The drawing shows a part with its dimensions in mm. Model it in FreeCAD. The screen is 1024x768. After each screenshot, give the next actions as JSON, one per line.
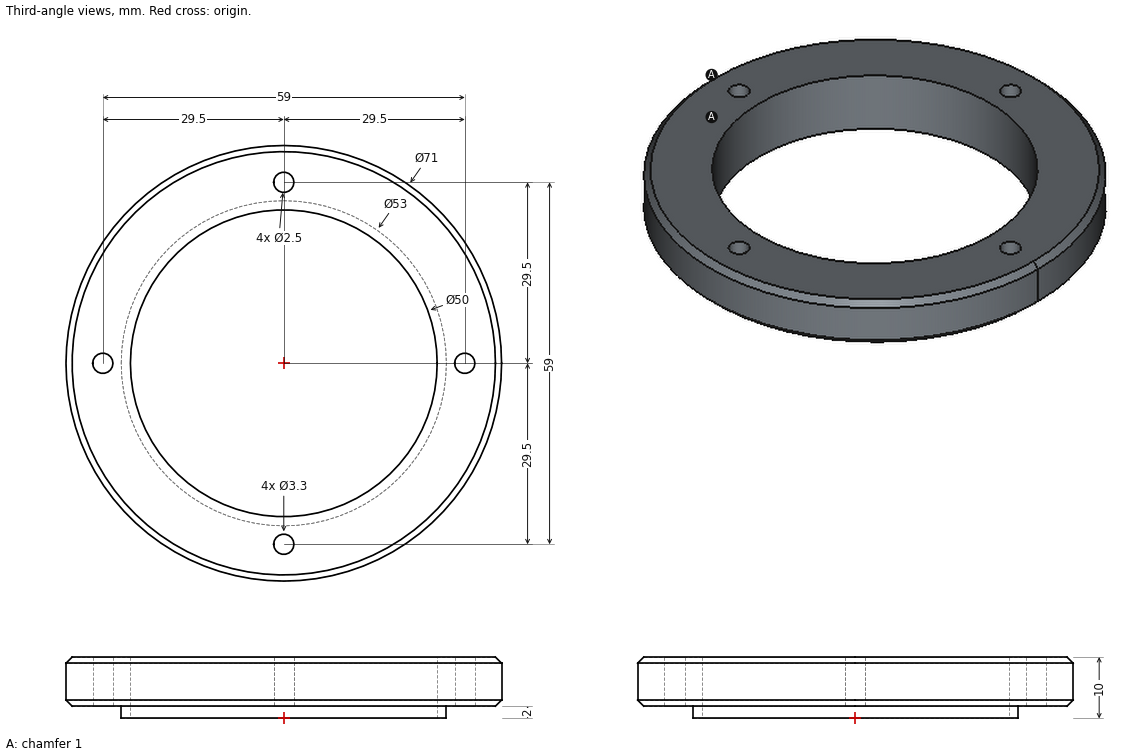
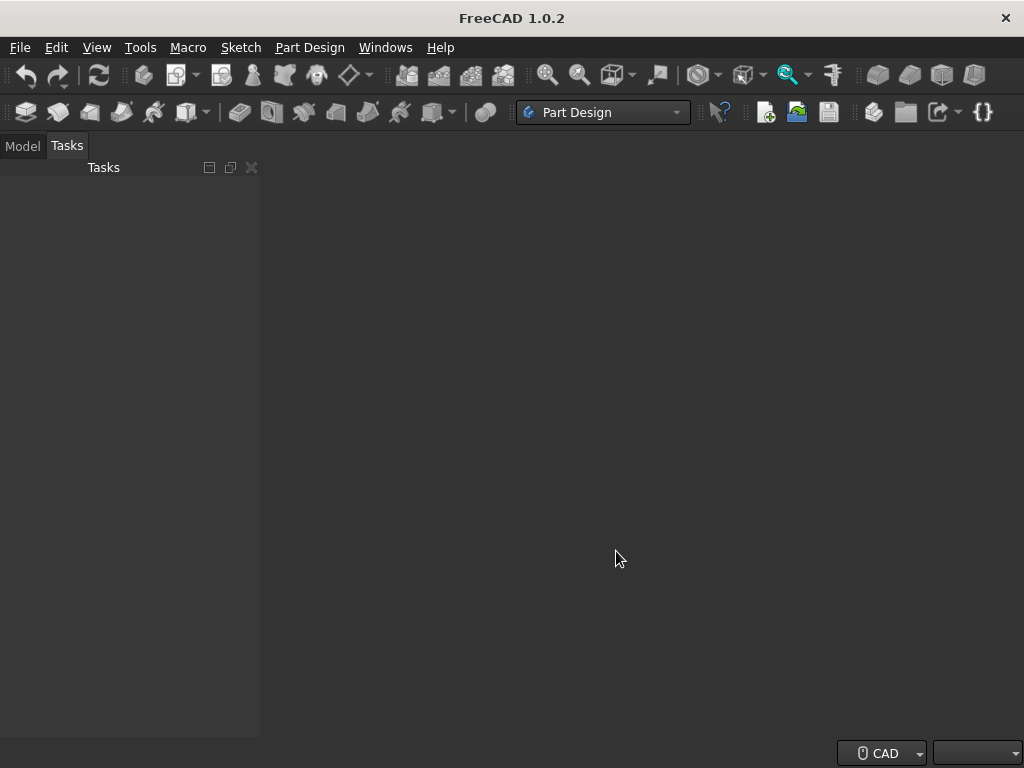
{"action": "left_click", "coordinate": [766, 112]}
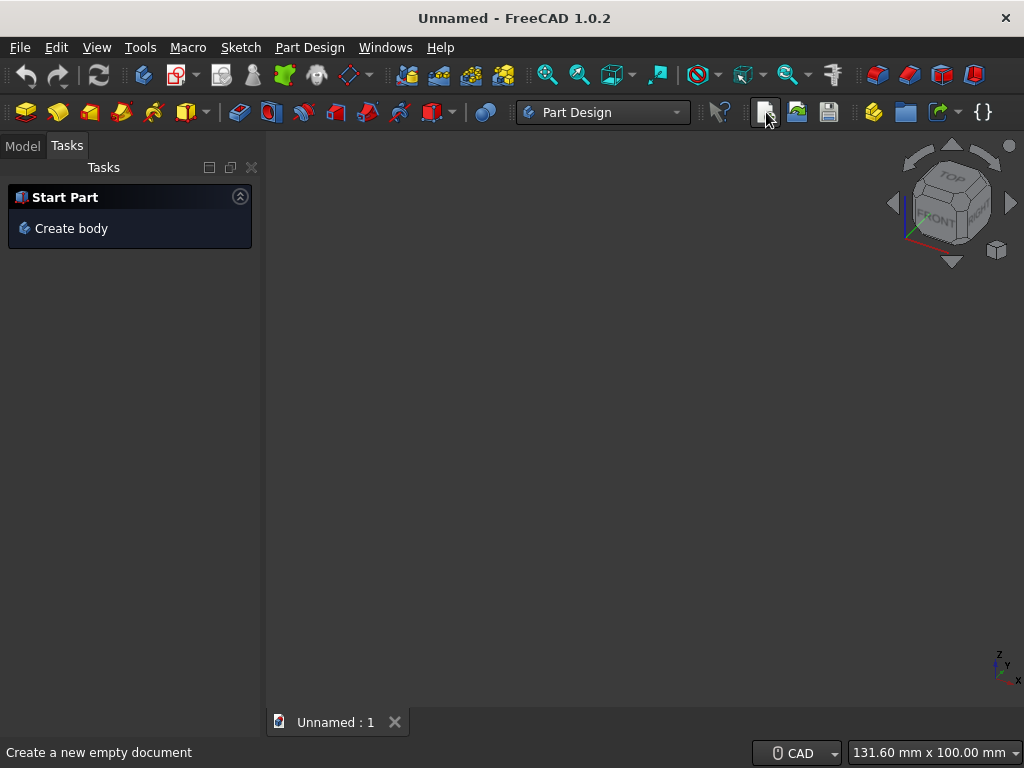
{"action": "left_click", "coordinate": [176, 76]}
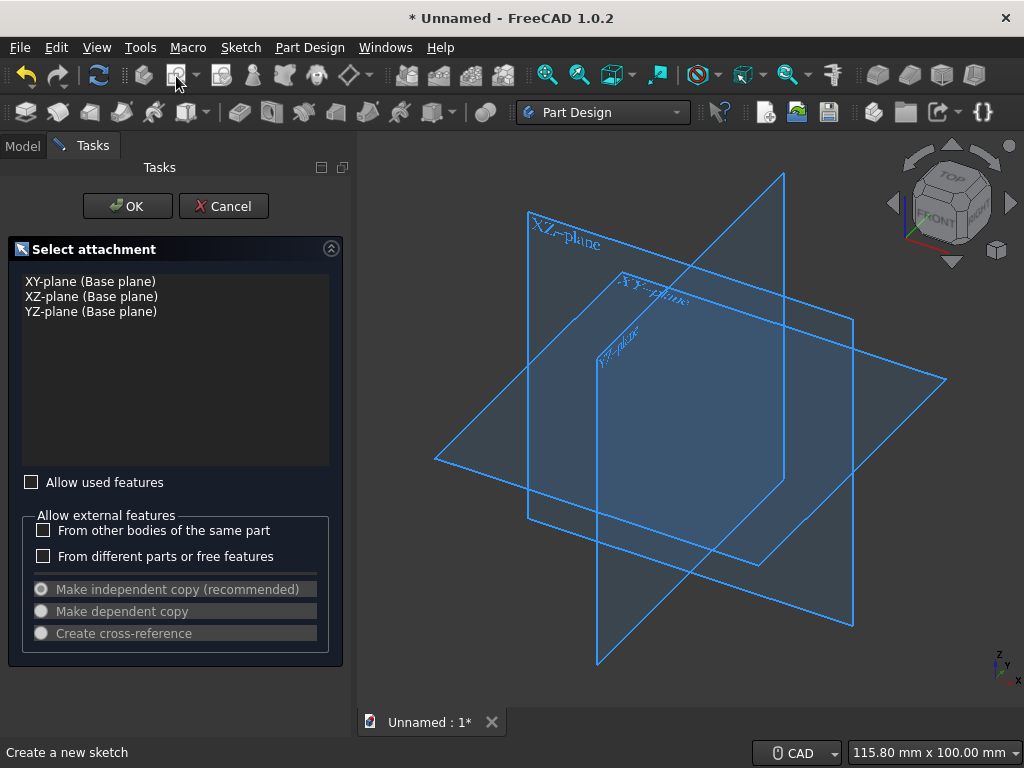
{"action": "left_click", "coordinate": [82, 282]}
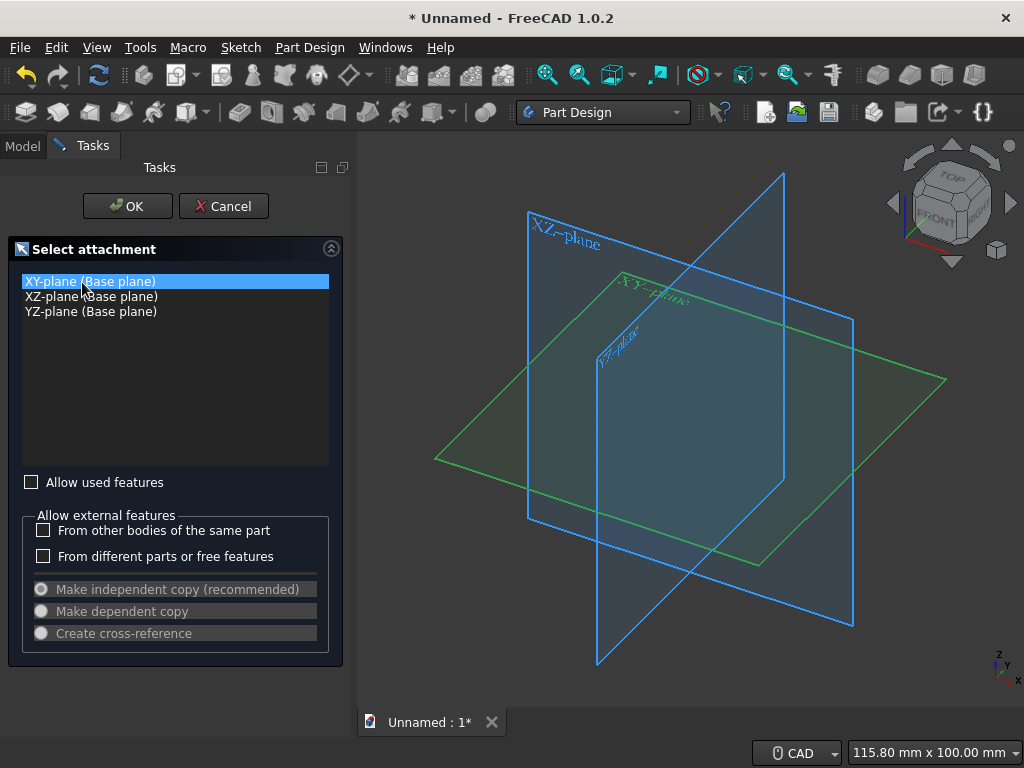
{"action": "left_click", "coordinate": [128, 206]}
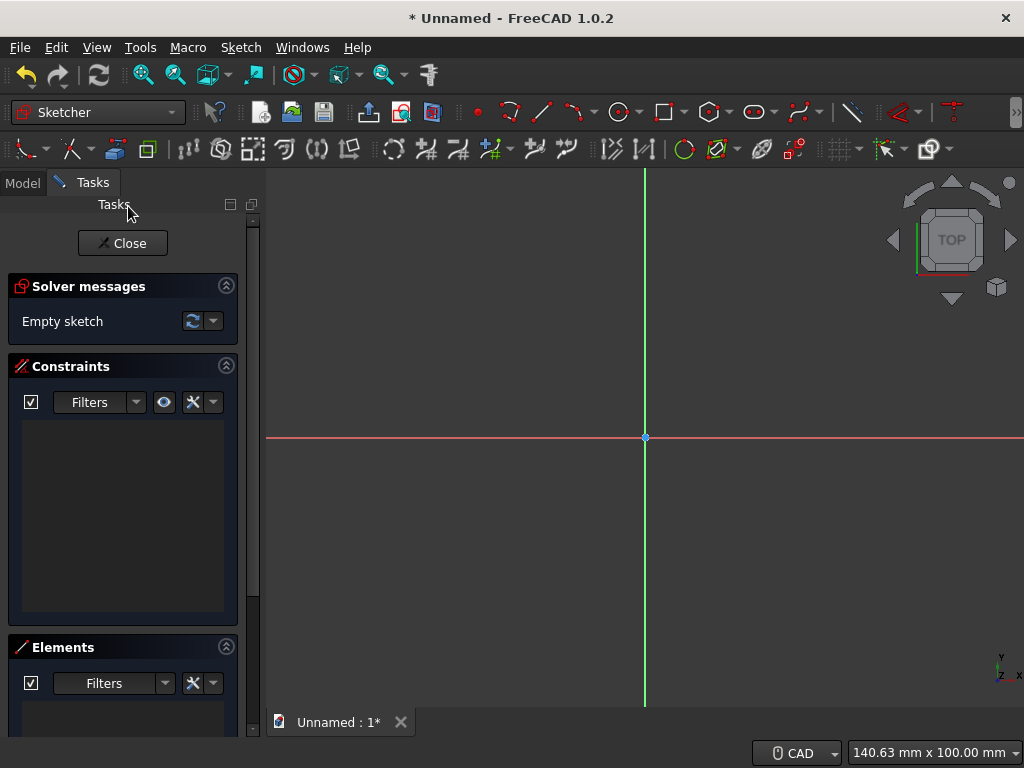
{"action": "scroll", "coordinate": [294, 437], "scroll_direction": "down", "scroll_amount": 1}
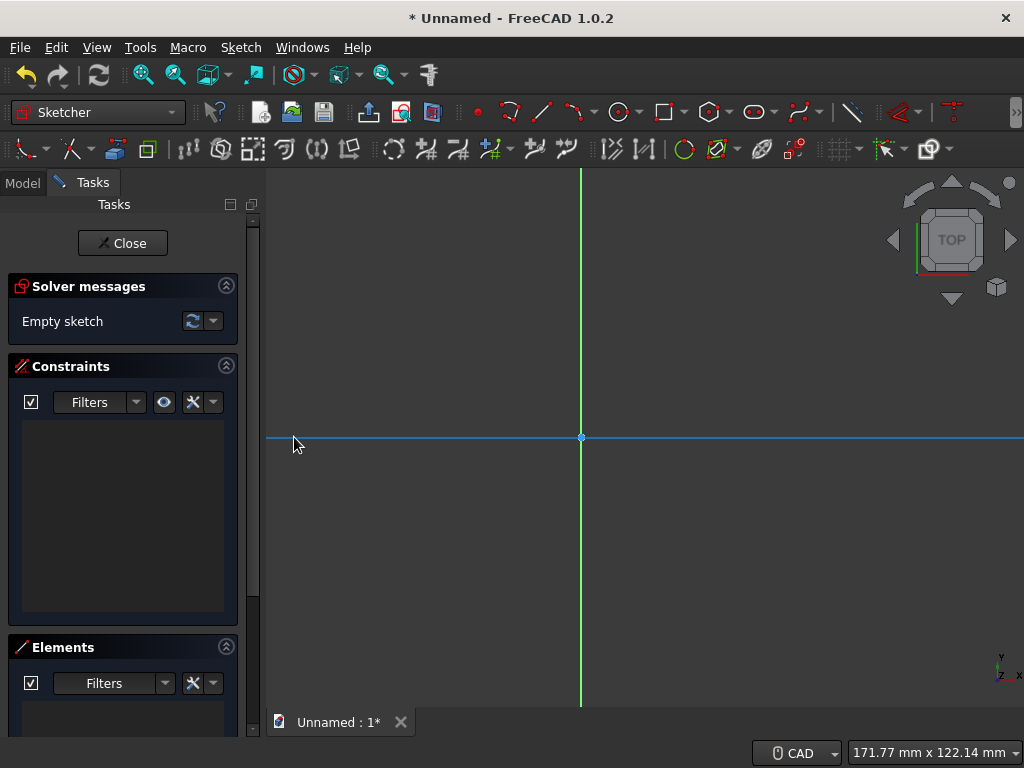
{"action": "key", "text": "g c"}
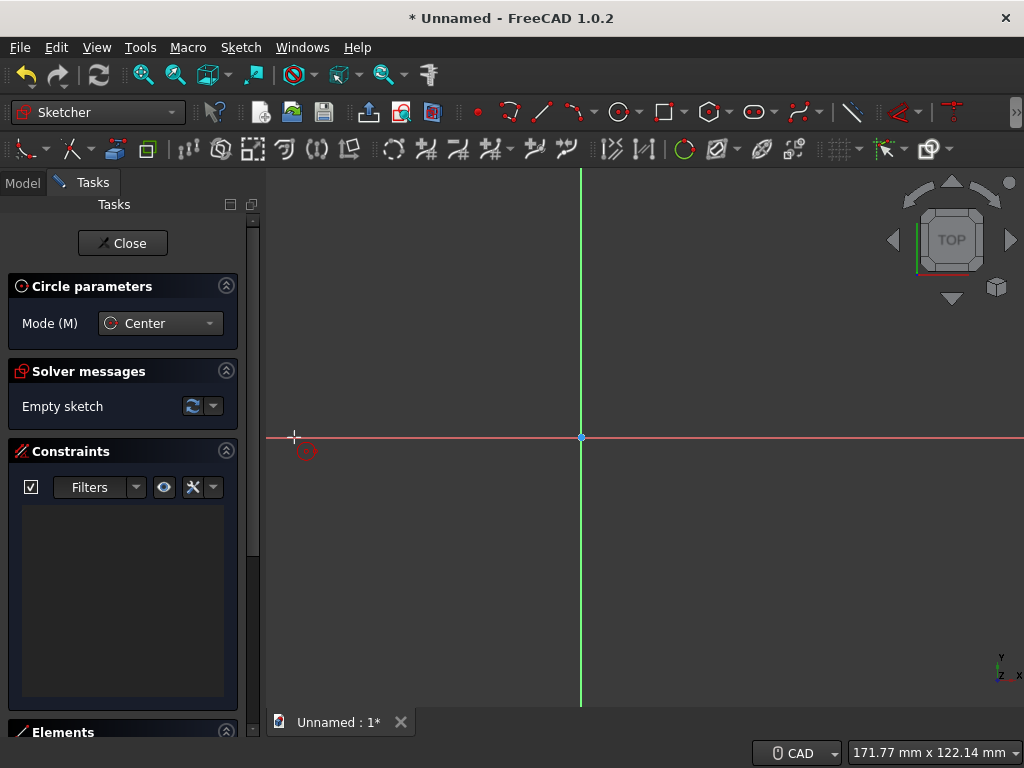
{"action": "left_click", "coordinate": [581, 438]}
{"action": "mouse_move", "coordinate": [692, 327]}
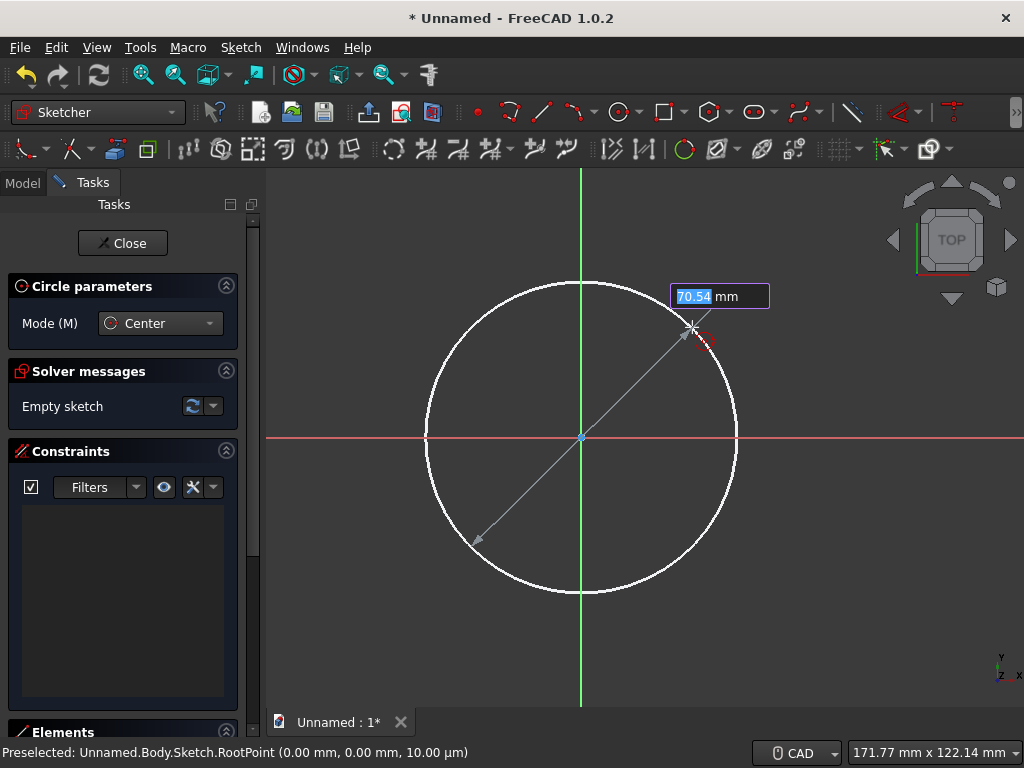
{"action": "type", "text": "71"}
{"action": "key", "text": "Return"}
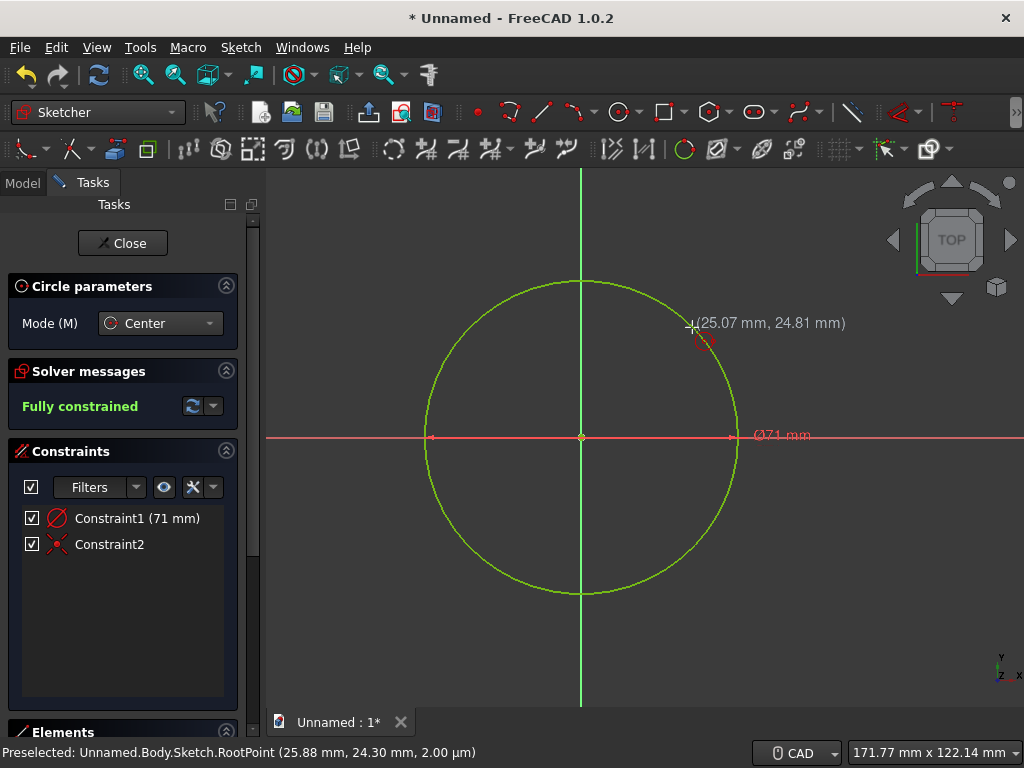
{"action": "left_click", "coordinate": [581, 438]}
{"action": "mouse_move", "coordinate": [659, 359]}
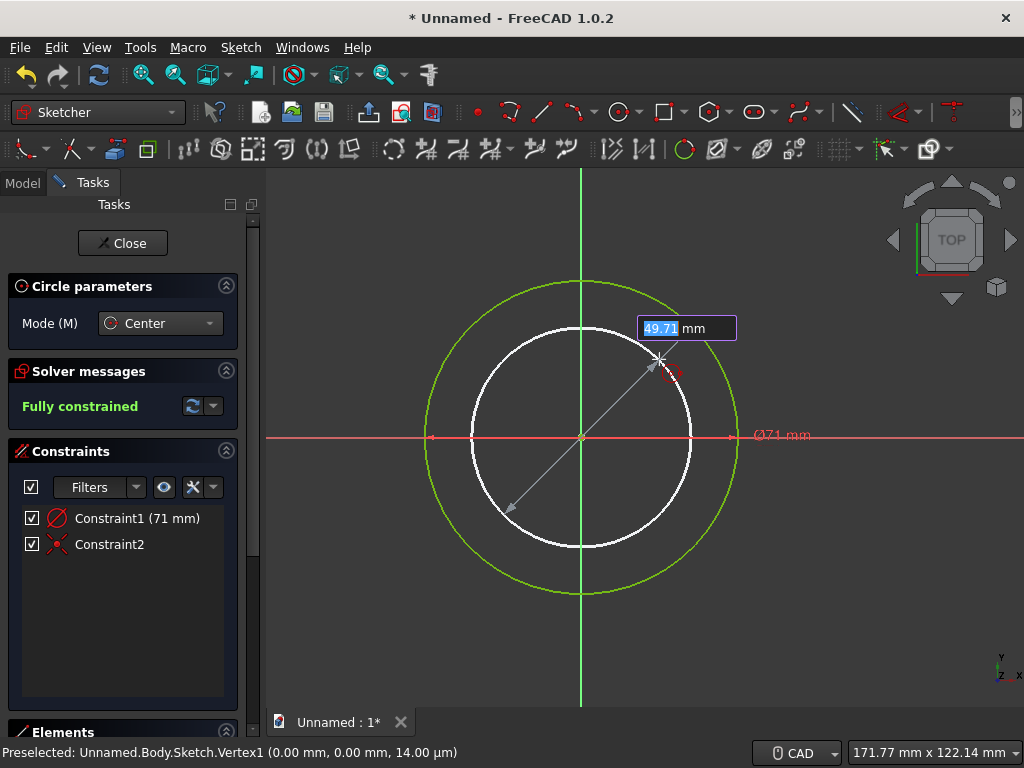
{"action": "type", "text": "50"}
{"action": "key", "text": "Return"}
{"action": "key", "text": "Escape"}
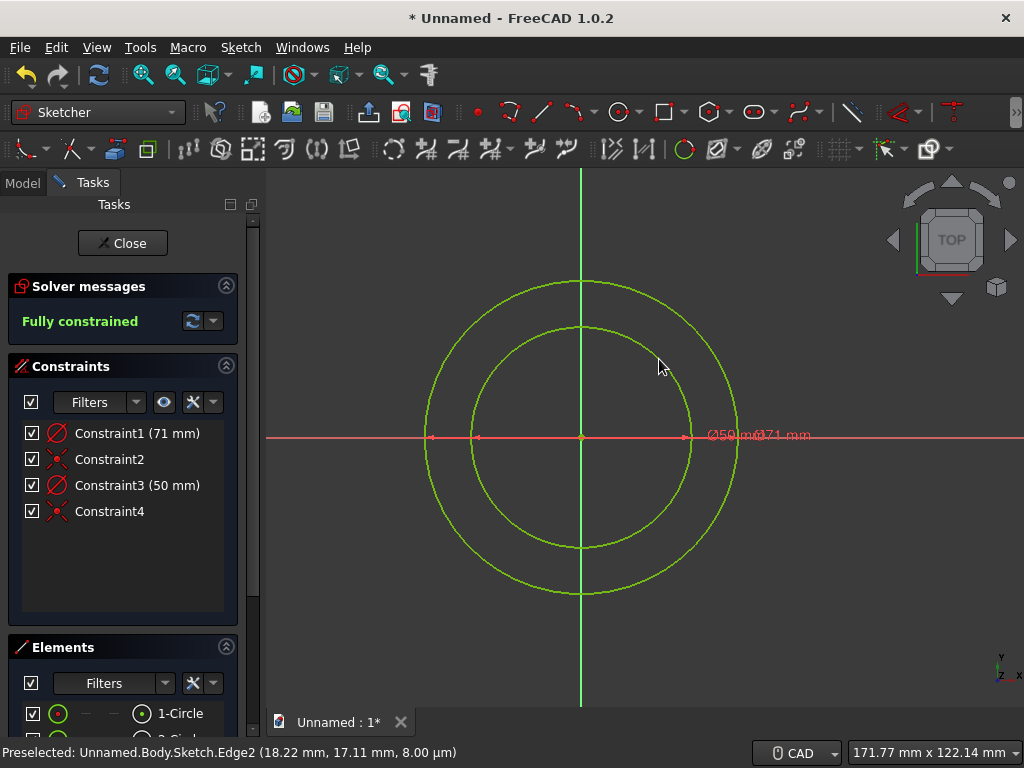
{"action": "left_click", "coordinate": [123, 243]}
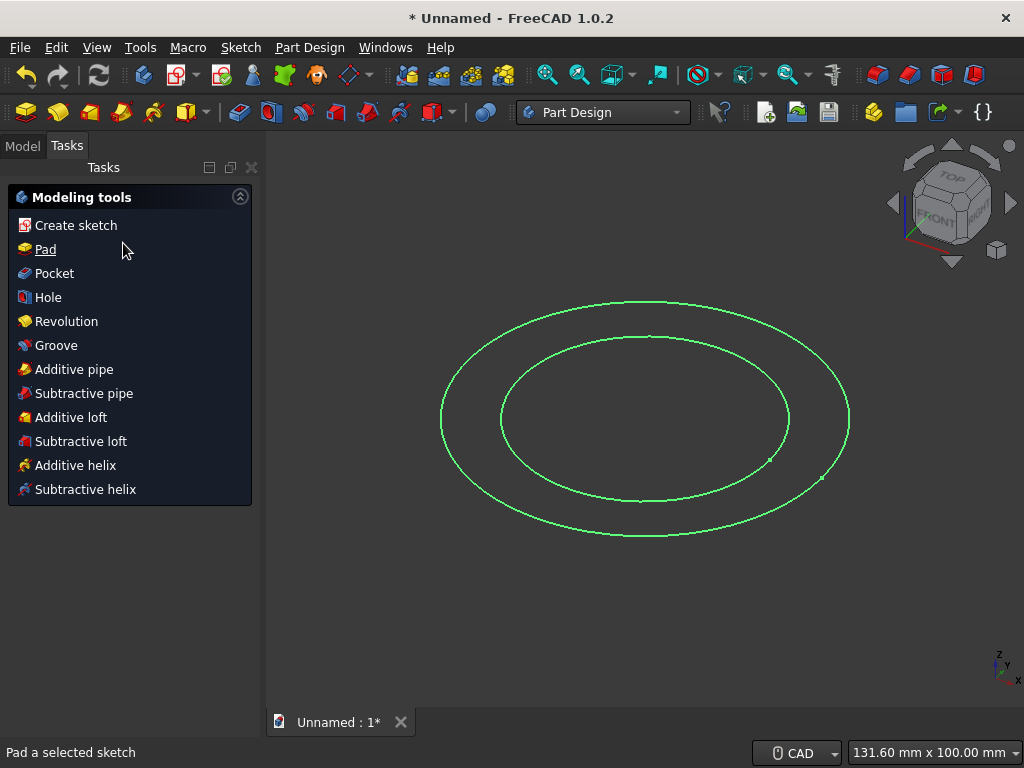
{"action": "left_click", "coordinate": [26, 112]}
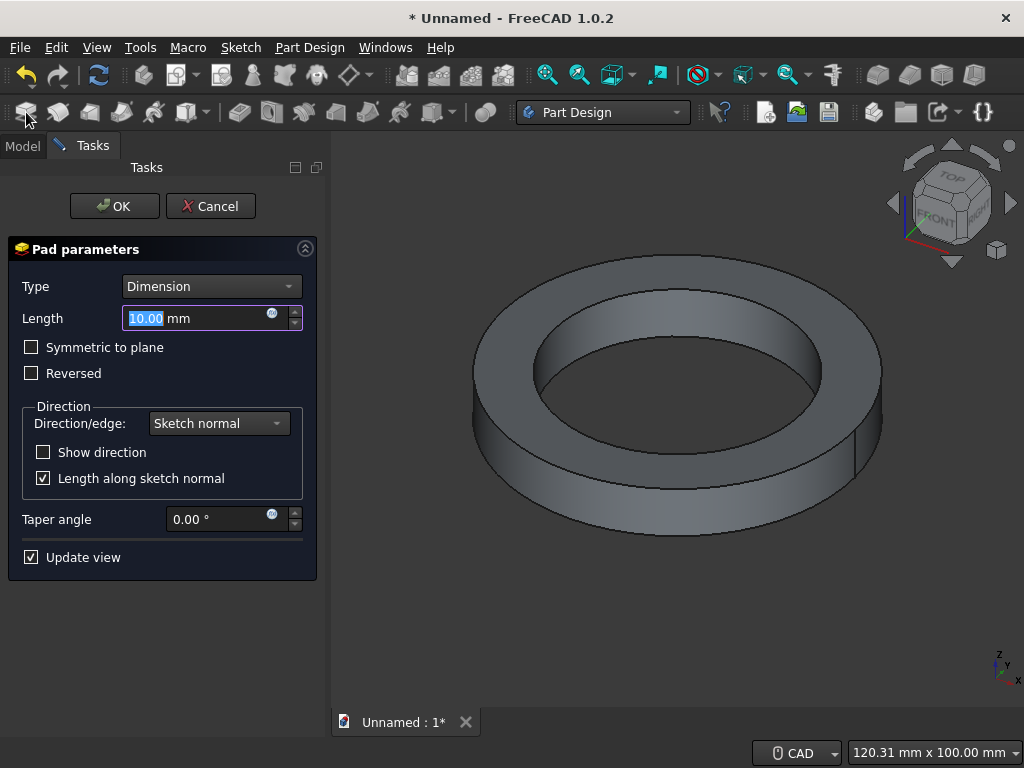
{"action": "type", "text": "10"}
{"action": "key", "text": "Tab"}